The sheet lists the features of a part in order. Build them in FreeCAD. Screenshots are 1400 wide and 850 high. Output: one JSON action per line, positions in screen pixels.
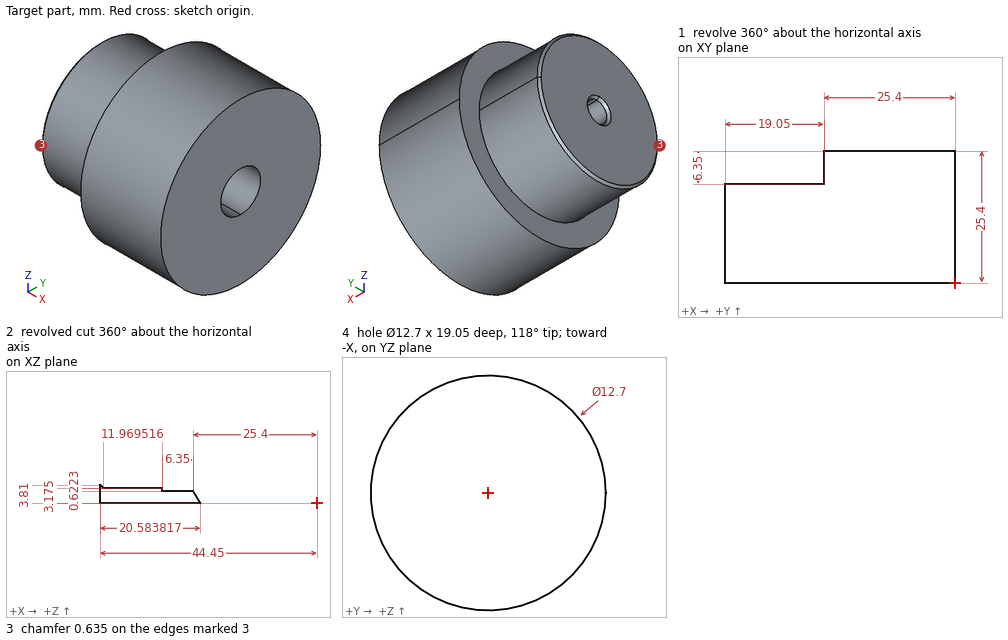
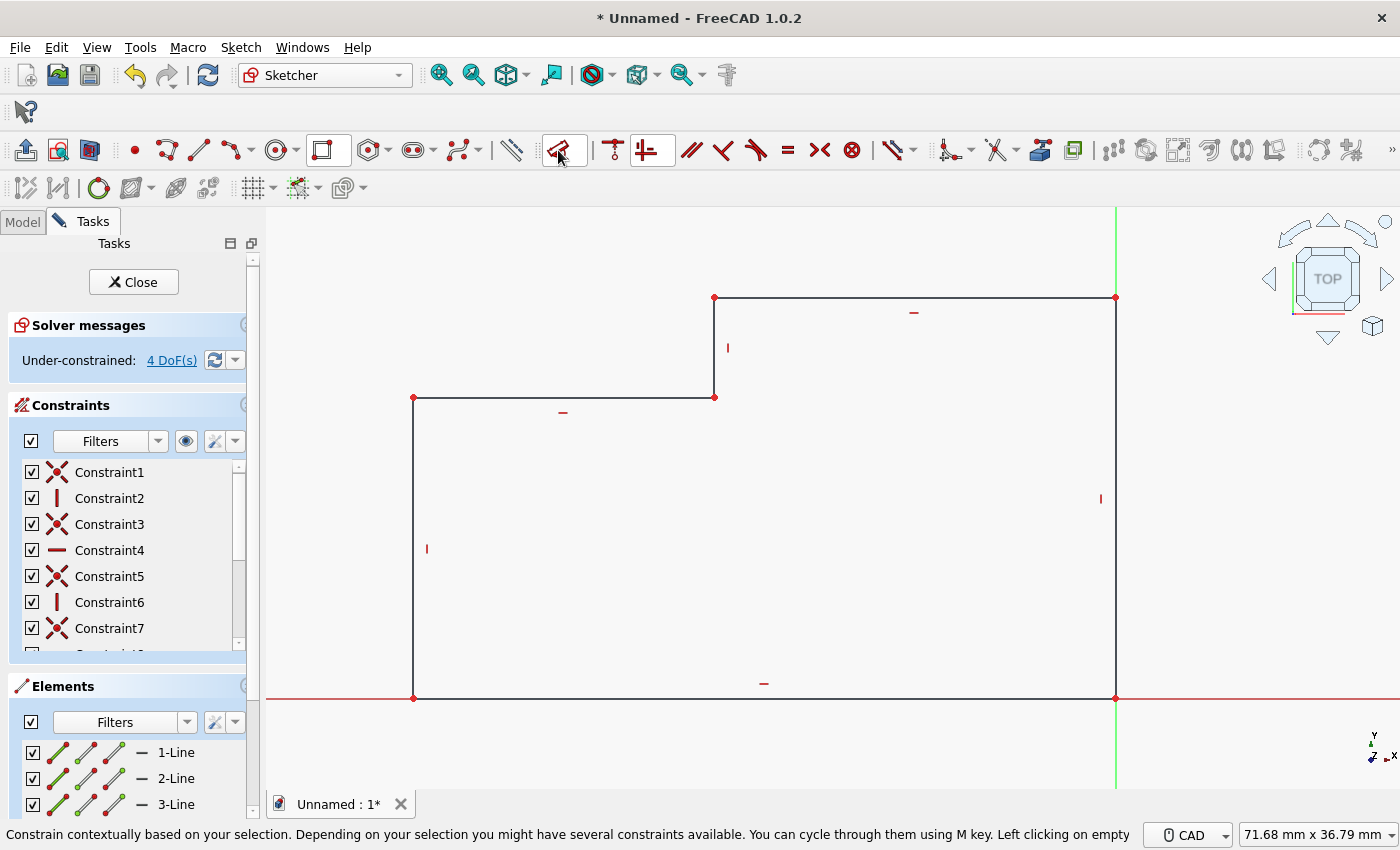
{"action": "left_click", "coordinate": [1116, 578]}
{"action": "left_click", "coordinate": [1150, 498]}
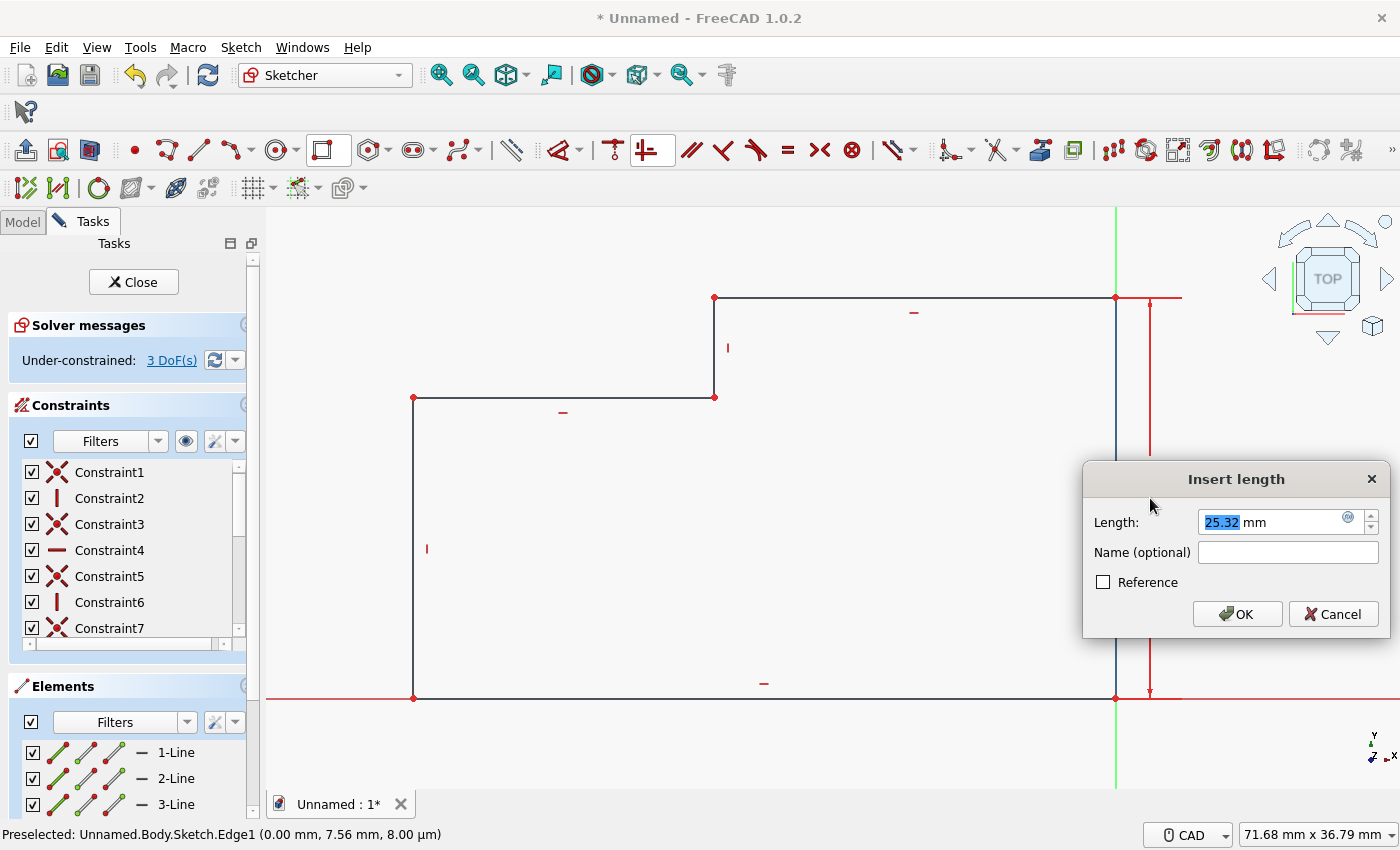
{"action": "type", "text": "25.4"}
{"action": "key", "text": "Return"}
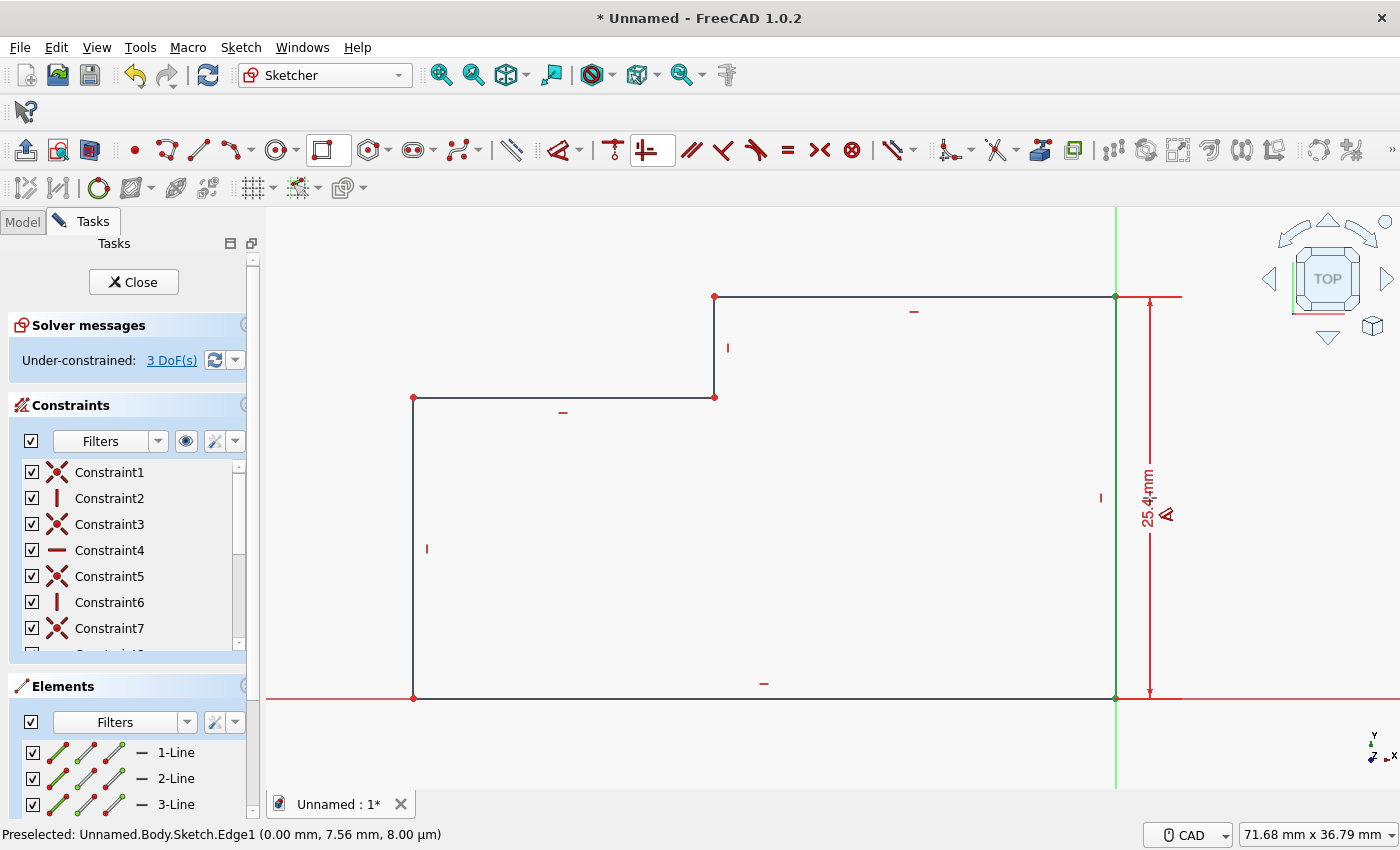
{"action": "left_click", "coordinate": [995, 297]}
{"action": "left_click", "coordinate": [915, 263]}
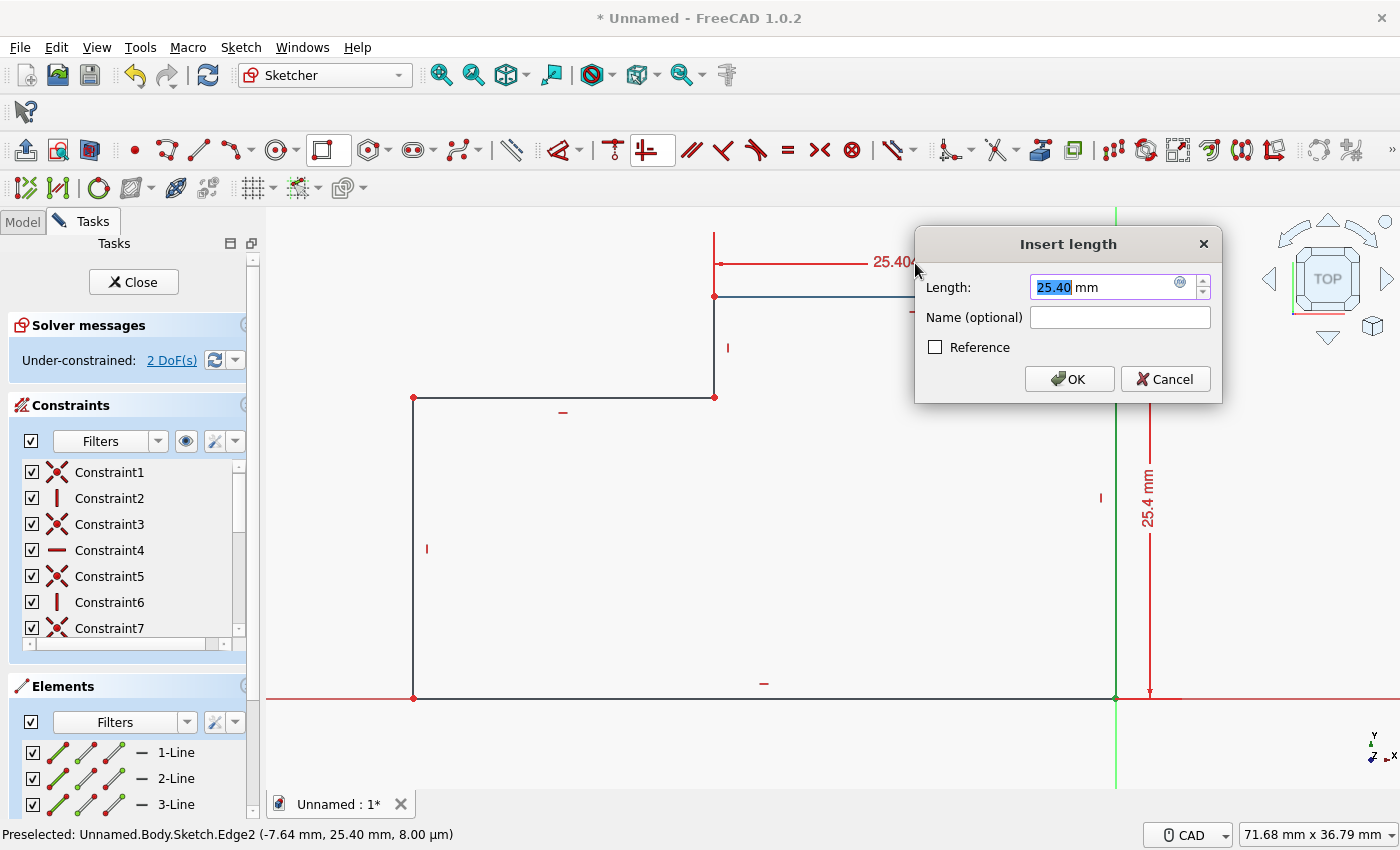
{"action": "type", "text": "25.4"}
{"action": "key", "text": "Return"}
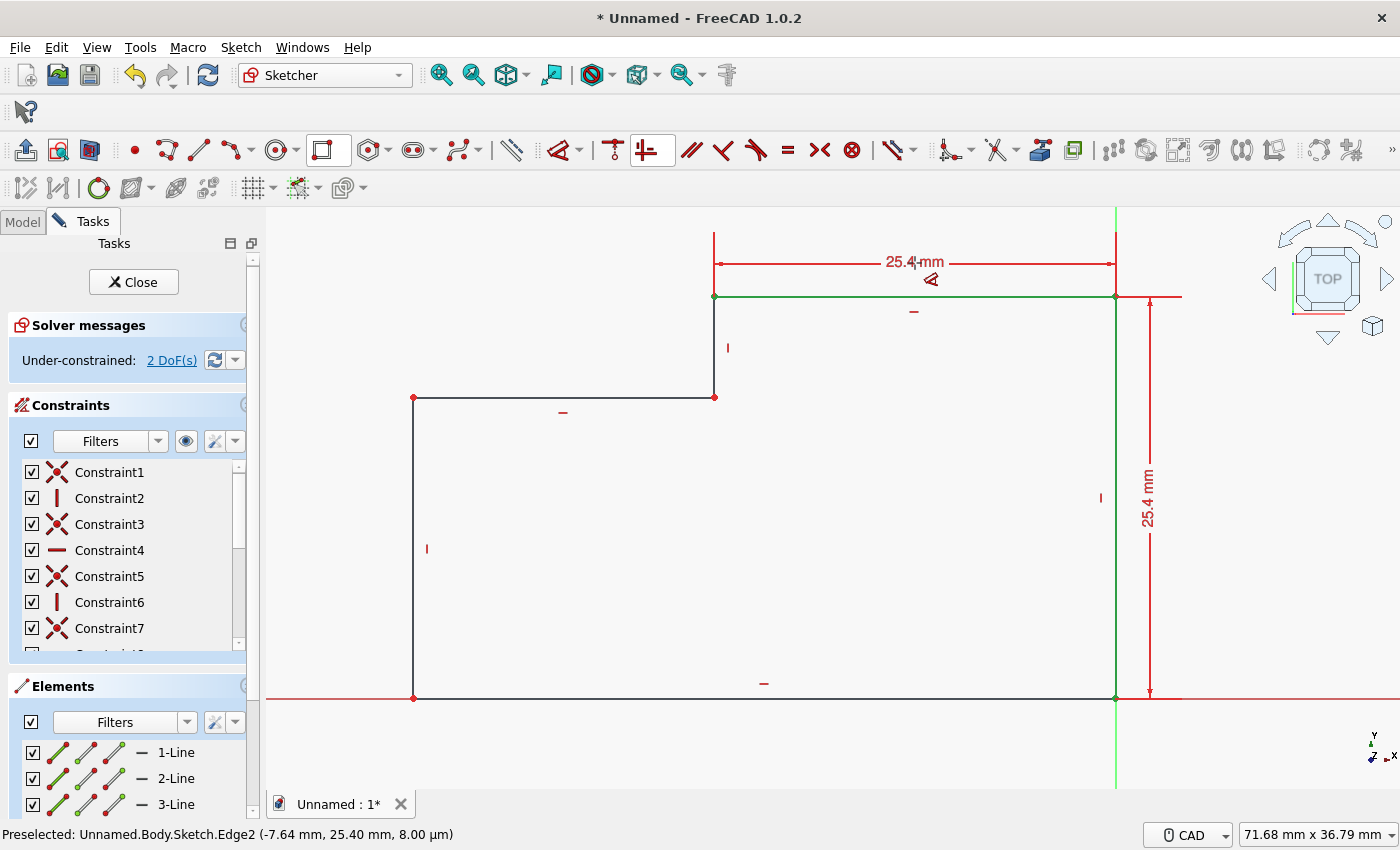
{"action": "left_click", "coordinate": [714, 327]}
{"action": "left_click", "coordinate": [680, 347]}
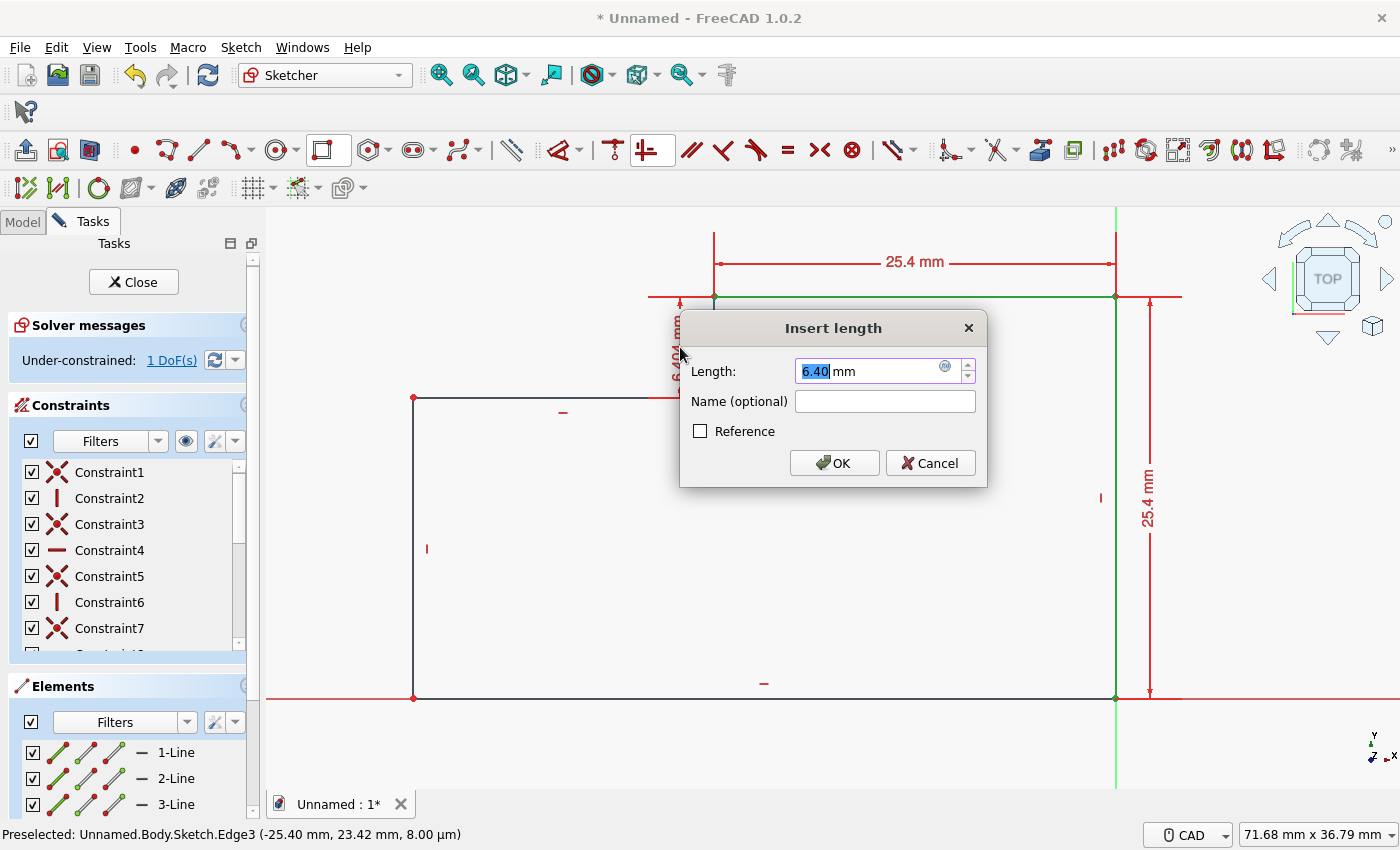
{"action": "type", "text": "6.35"}
{"action": "key", "text": "Return"}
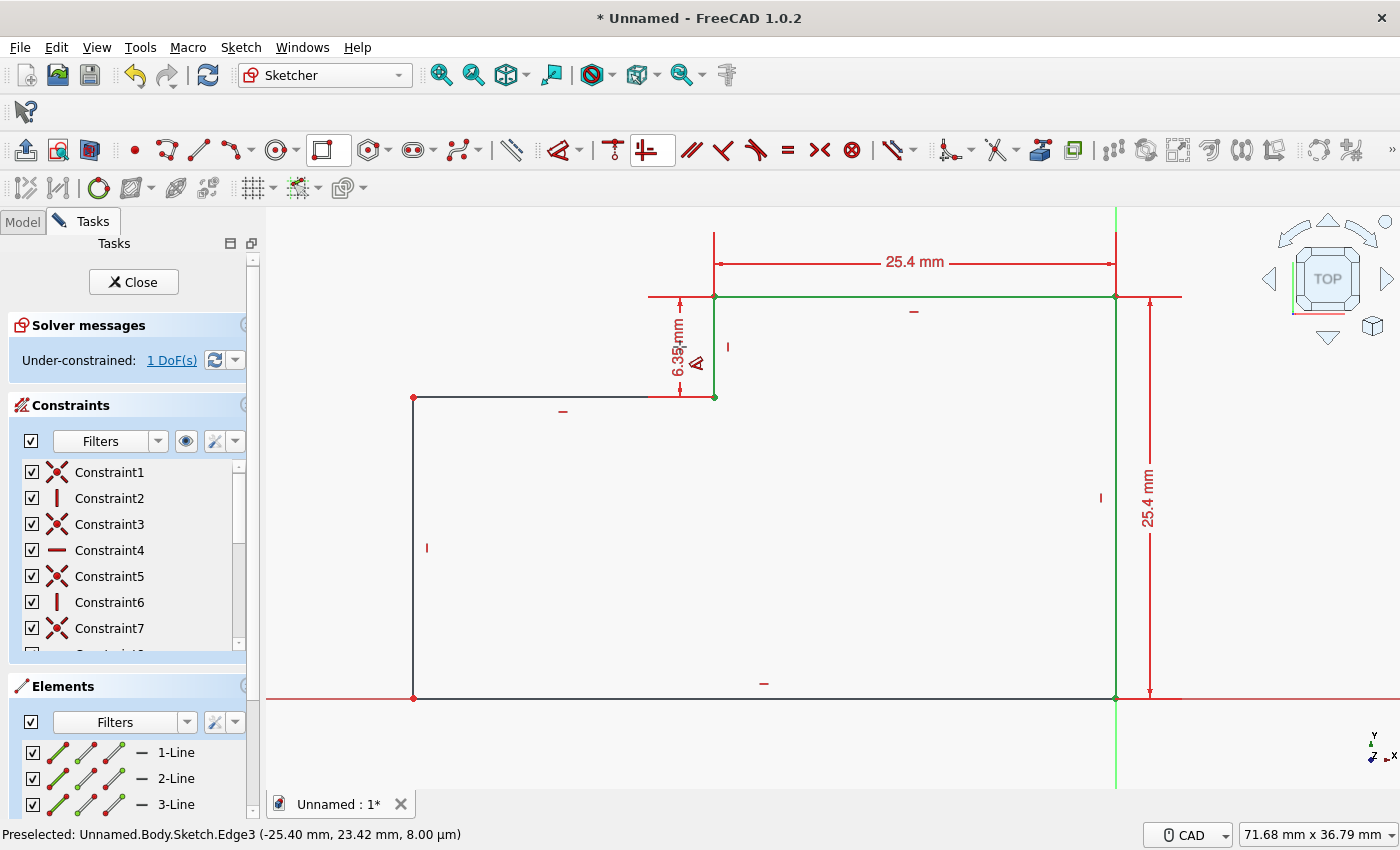
{"action": "left_click", "coordinate": [624, 397]}
{"action": "left_click", "coordinate": [564, 363]}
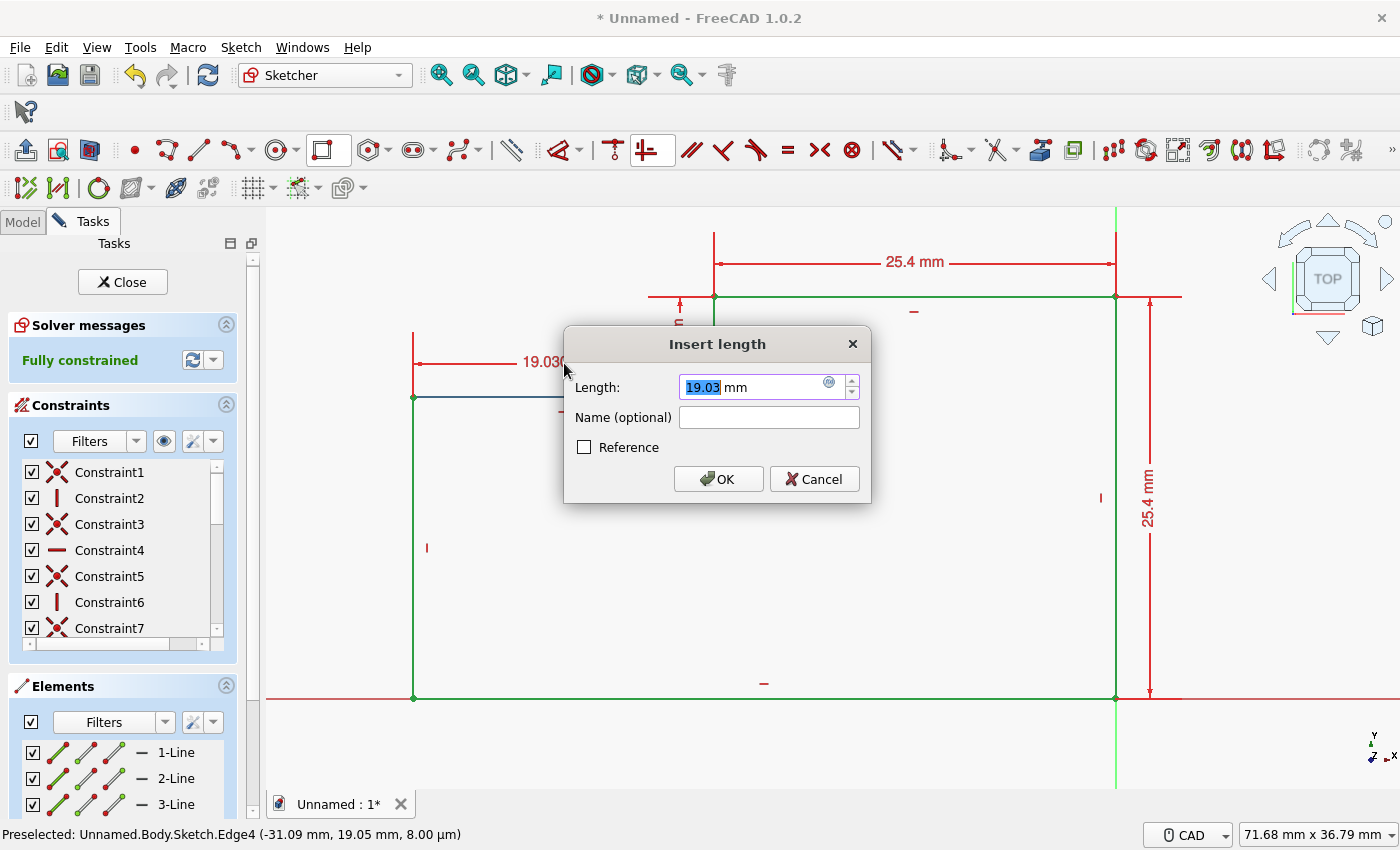
{"action": "type", "text": "19.05"}
{"action": "key", "text": "Return"}
{"action": "key", "text": "Escape"}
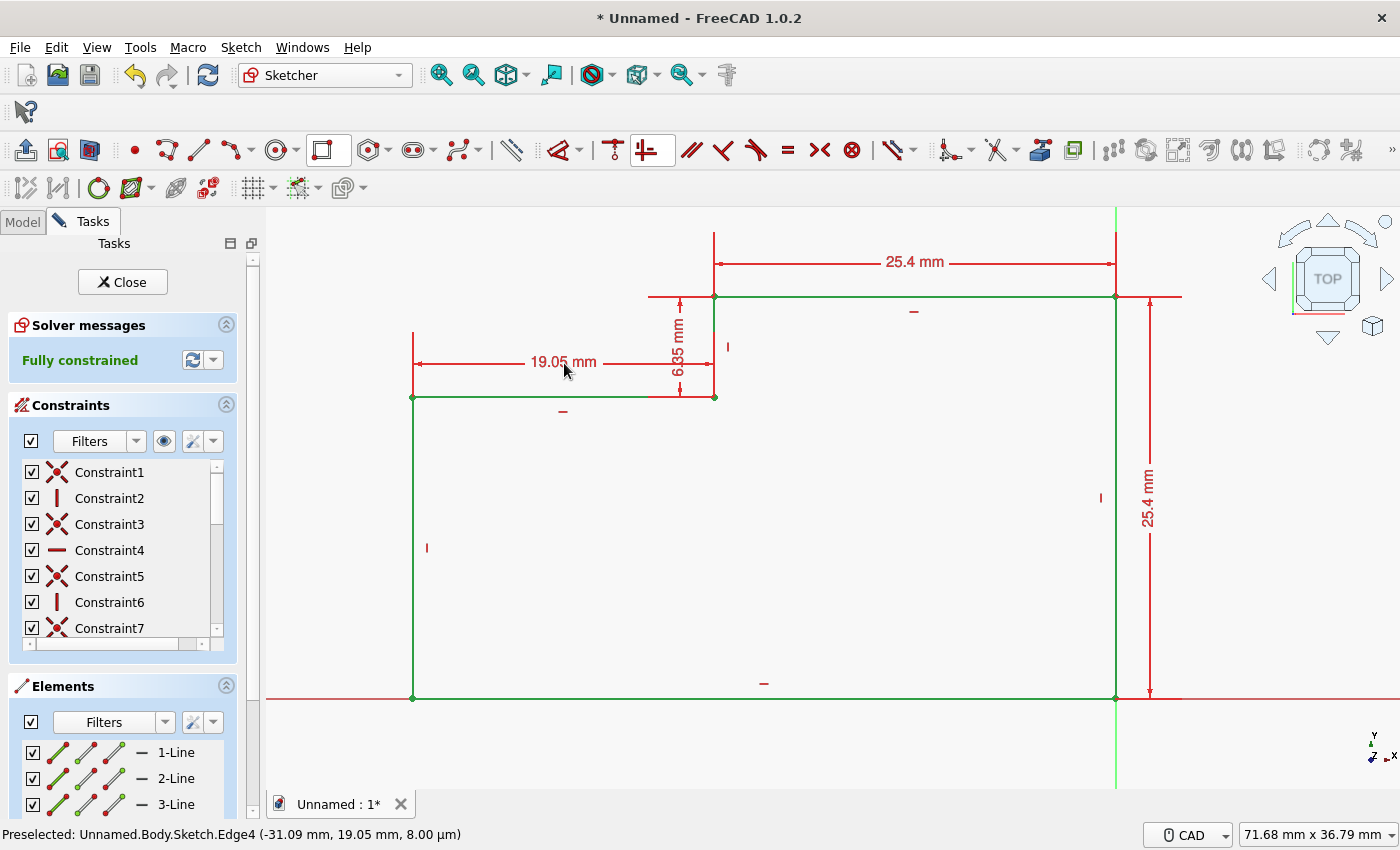
{"action": "left_click", "coordinate": [123, 282]}